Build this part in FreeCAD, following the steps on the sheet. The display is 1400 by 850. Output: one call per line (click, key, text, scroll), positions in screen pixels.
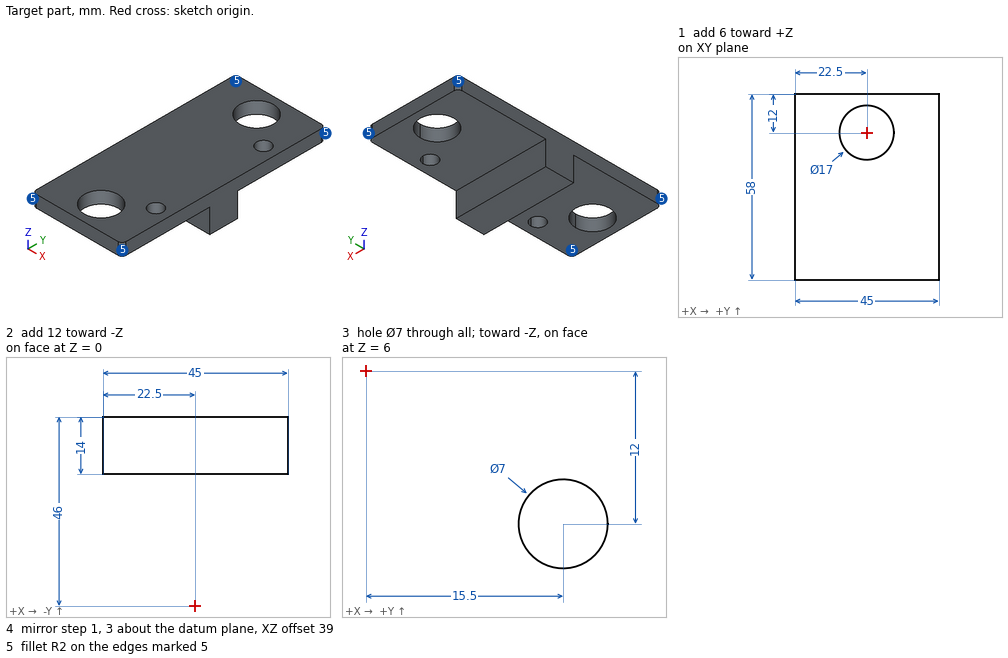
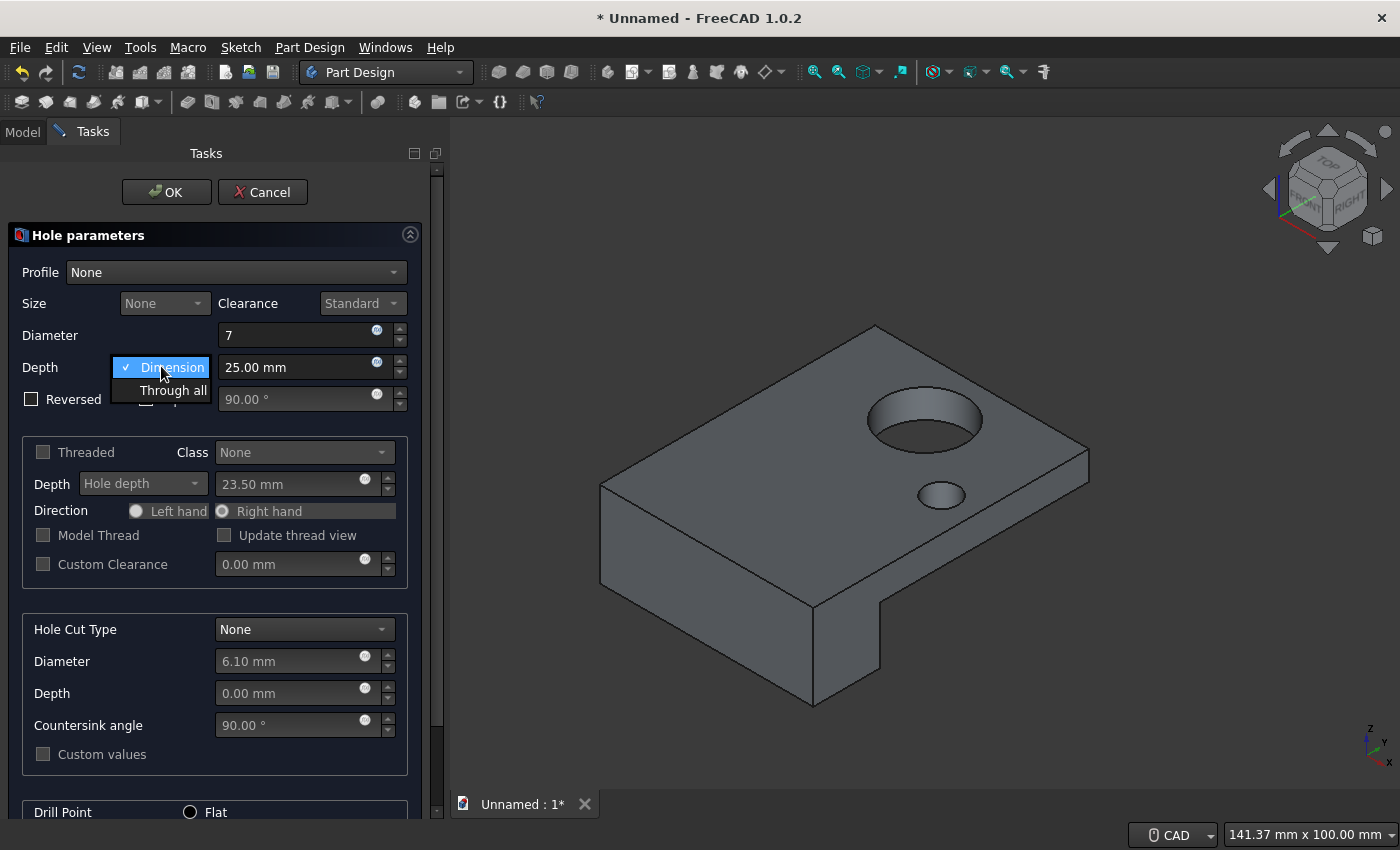
click(160, 390)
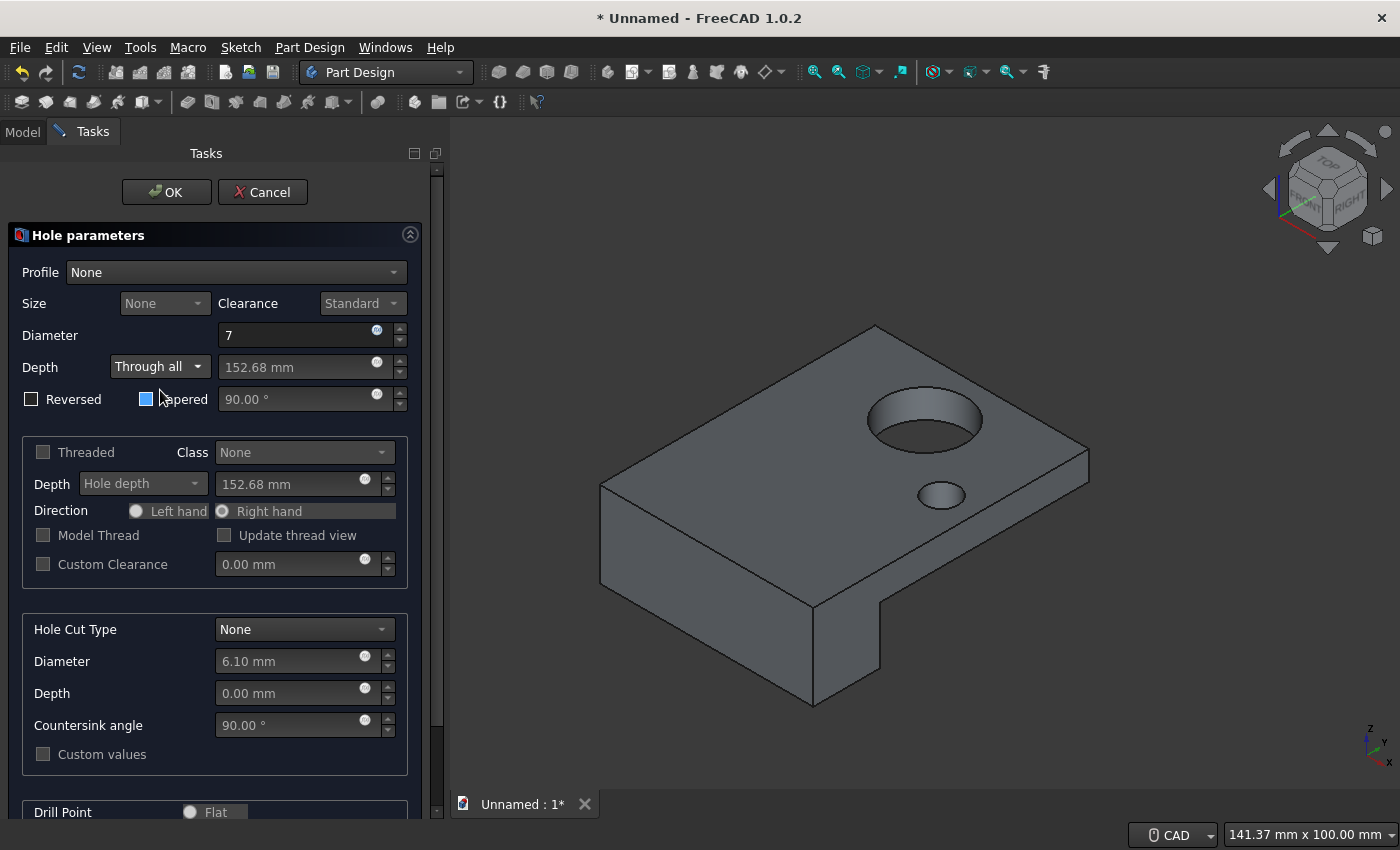
click(167, 192)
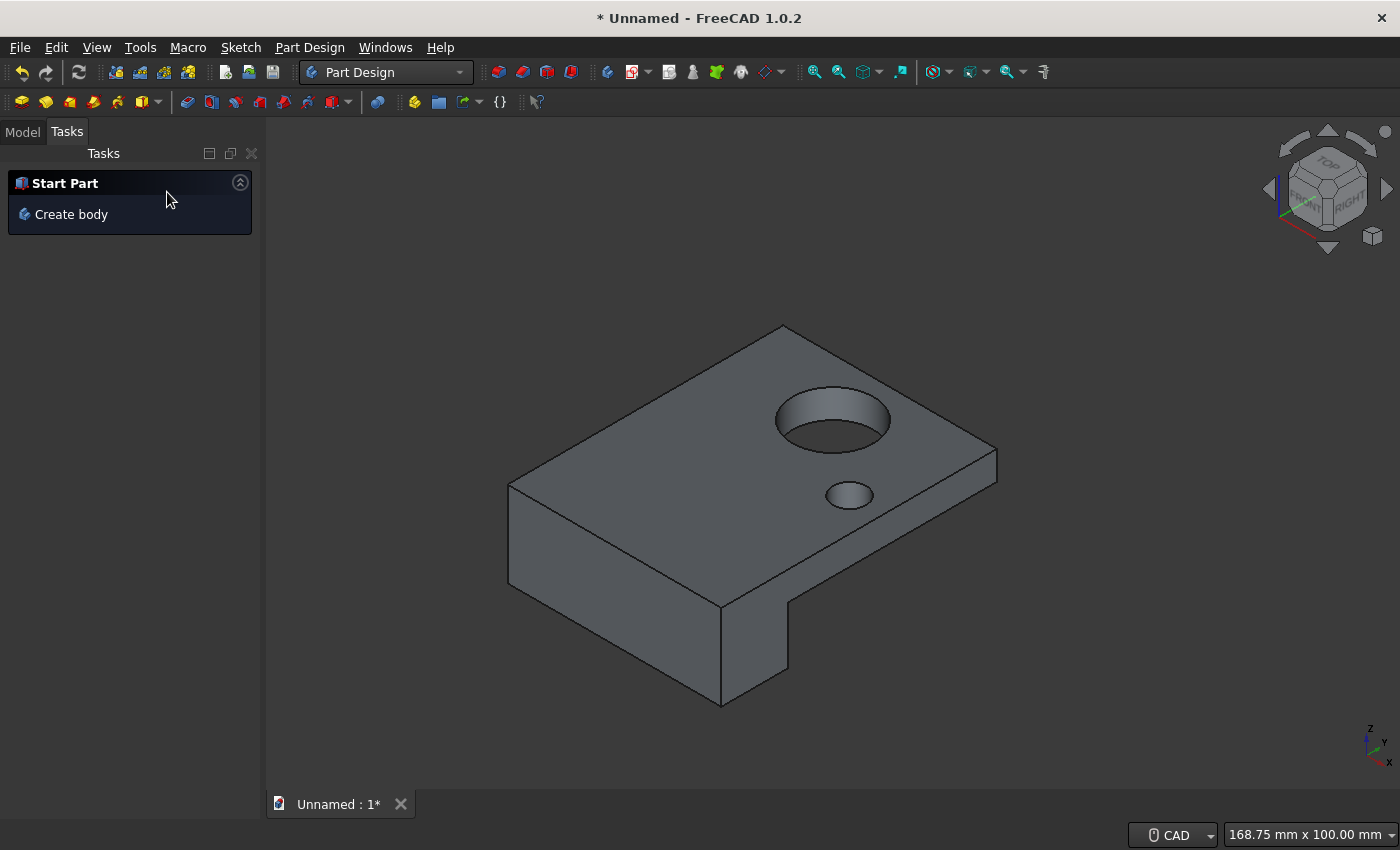
click(23, 131)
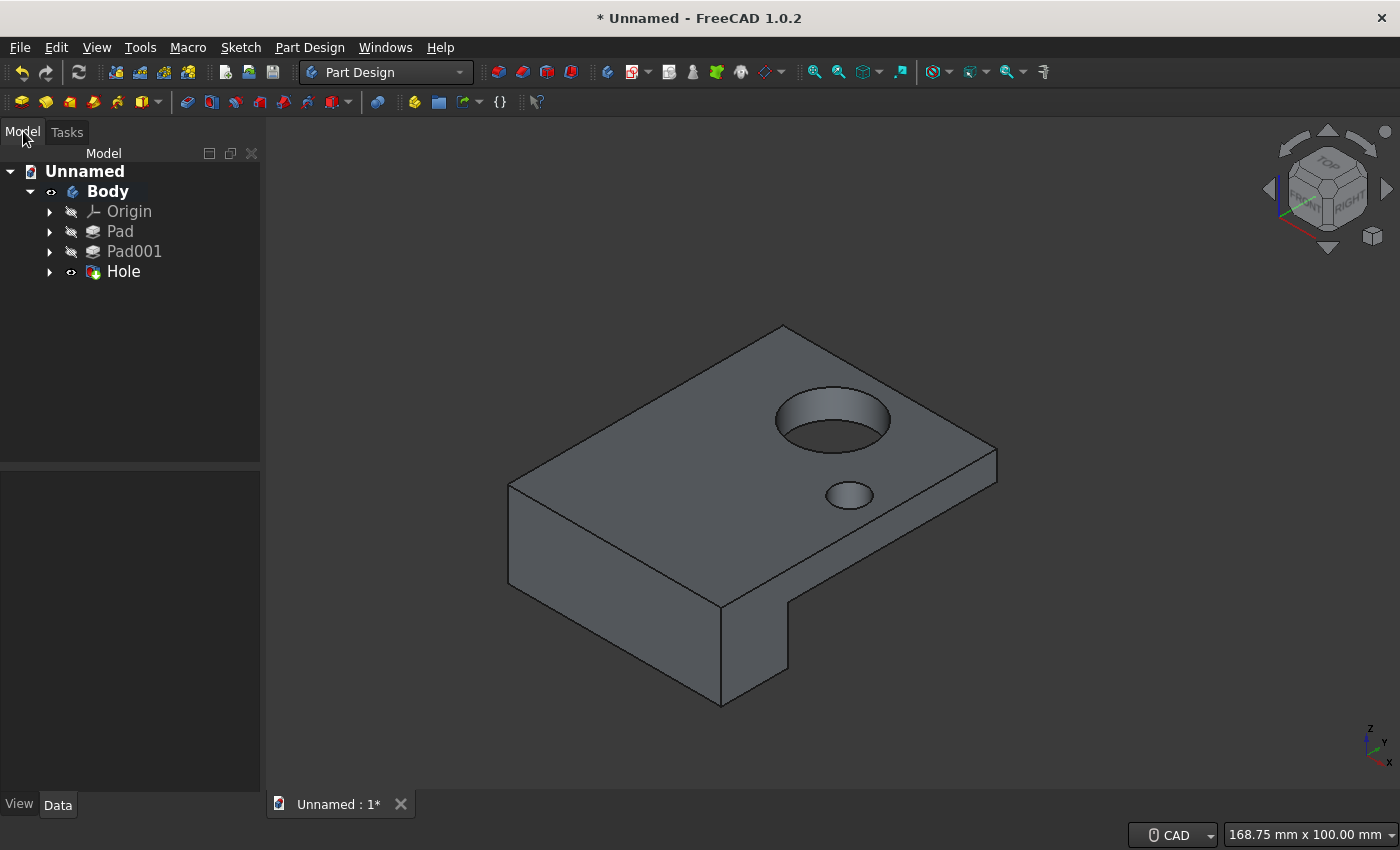
click(50, 212)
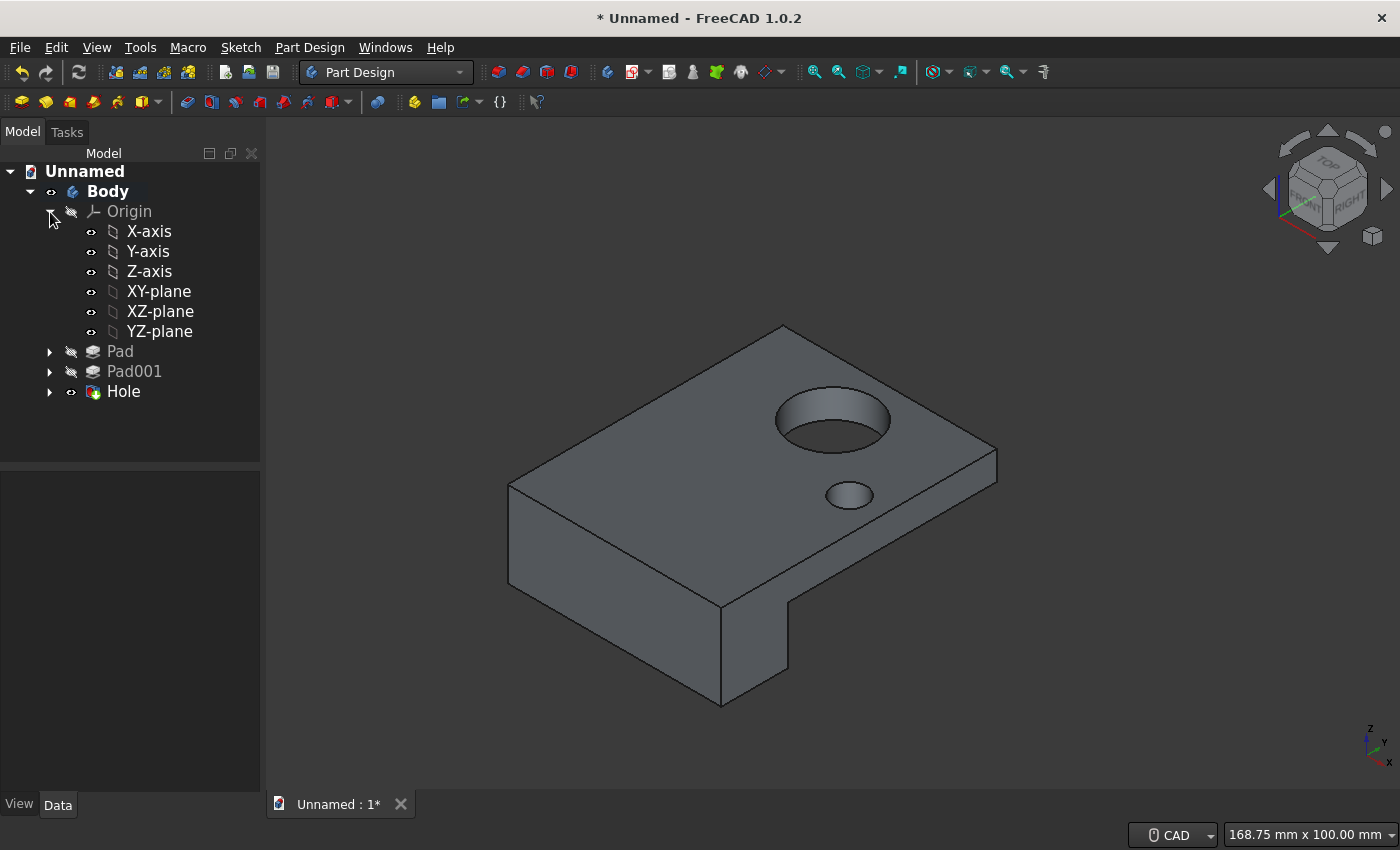
click(136, 312)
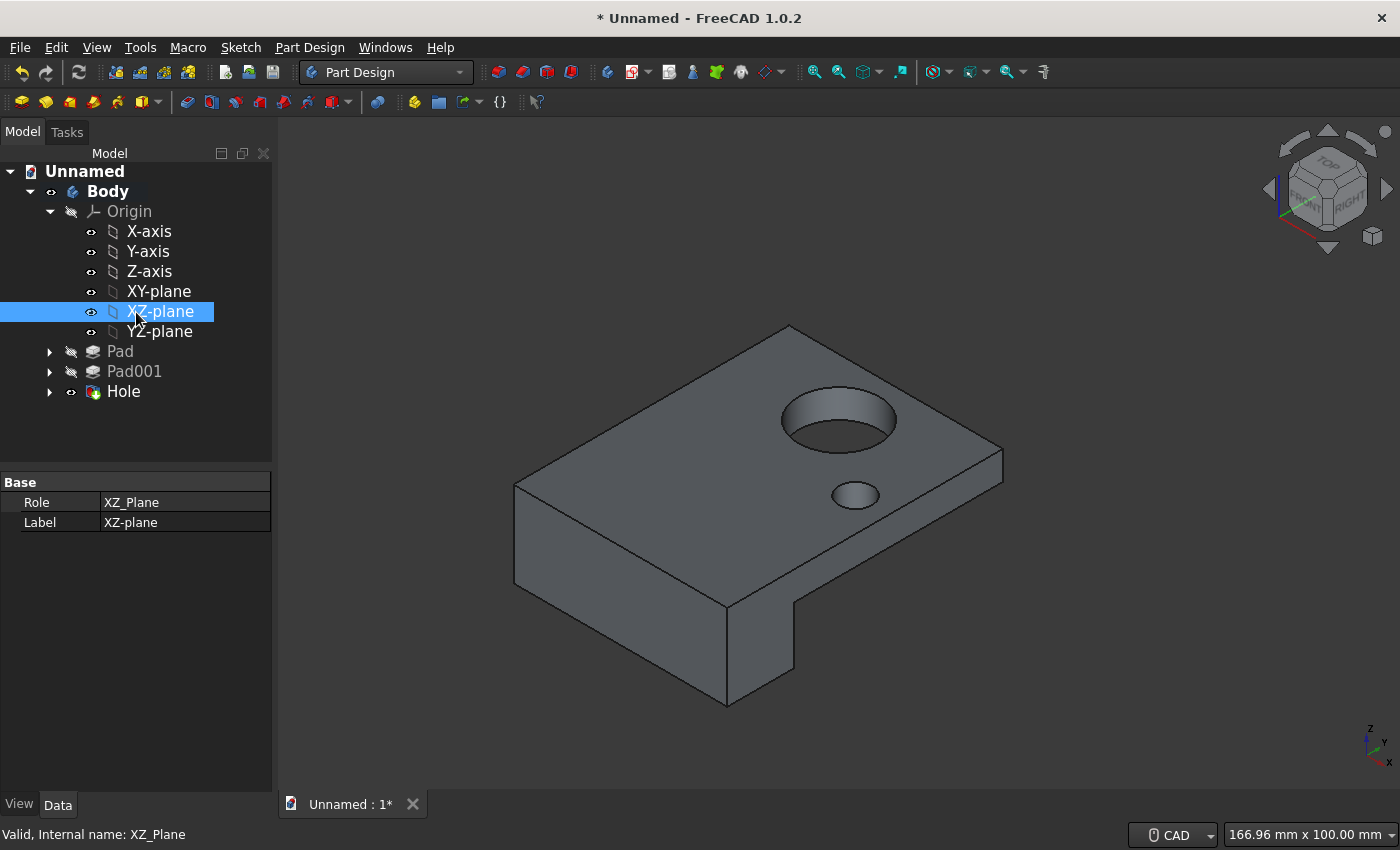
click(766, 72)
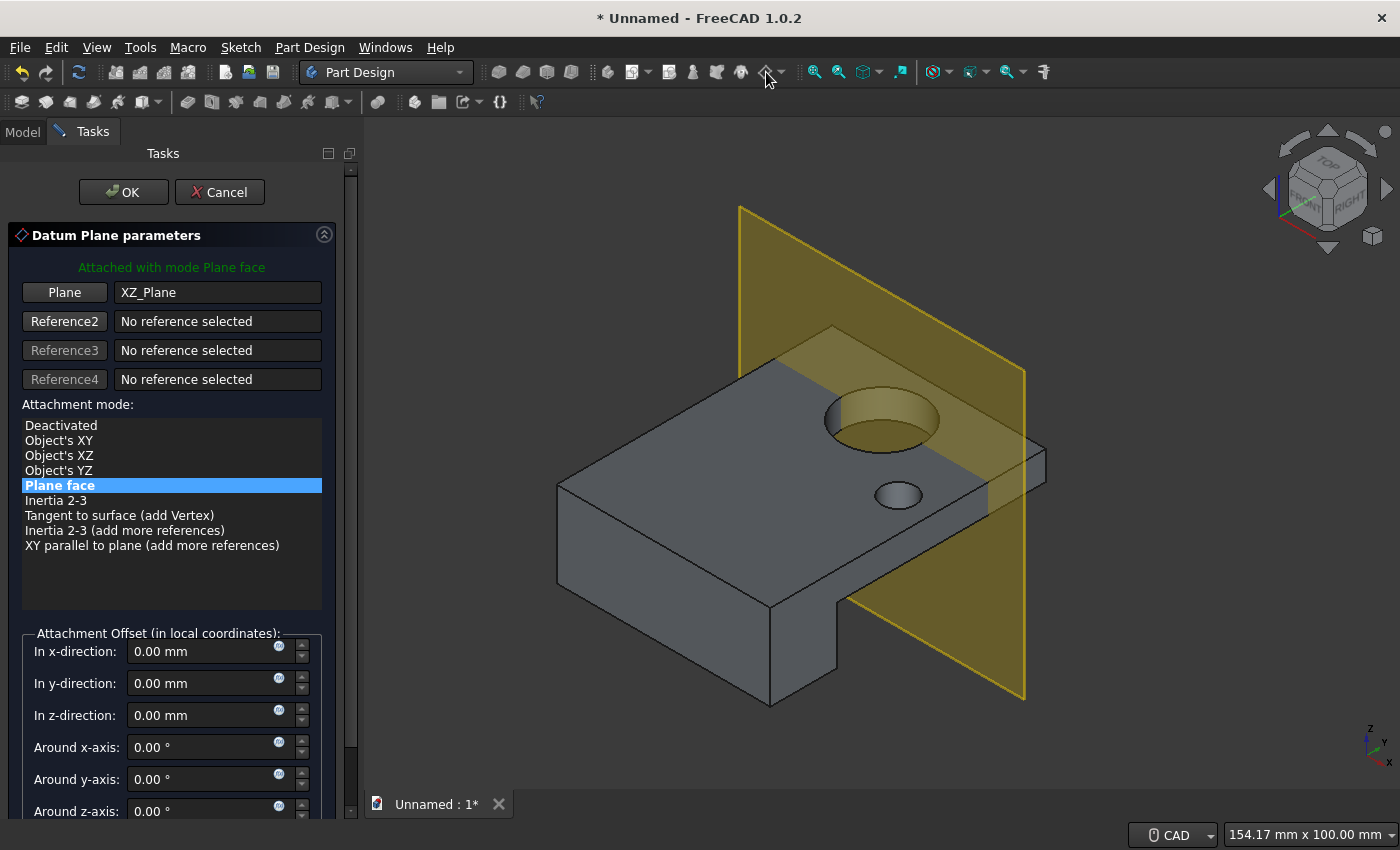
triple_click(210, 715)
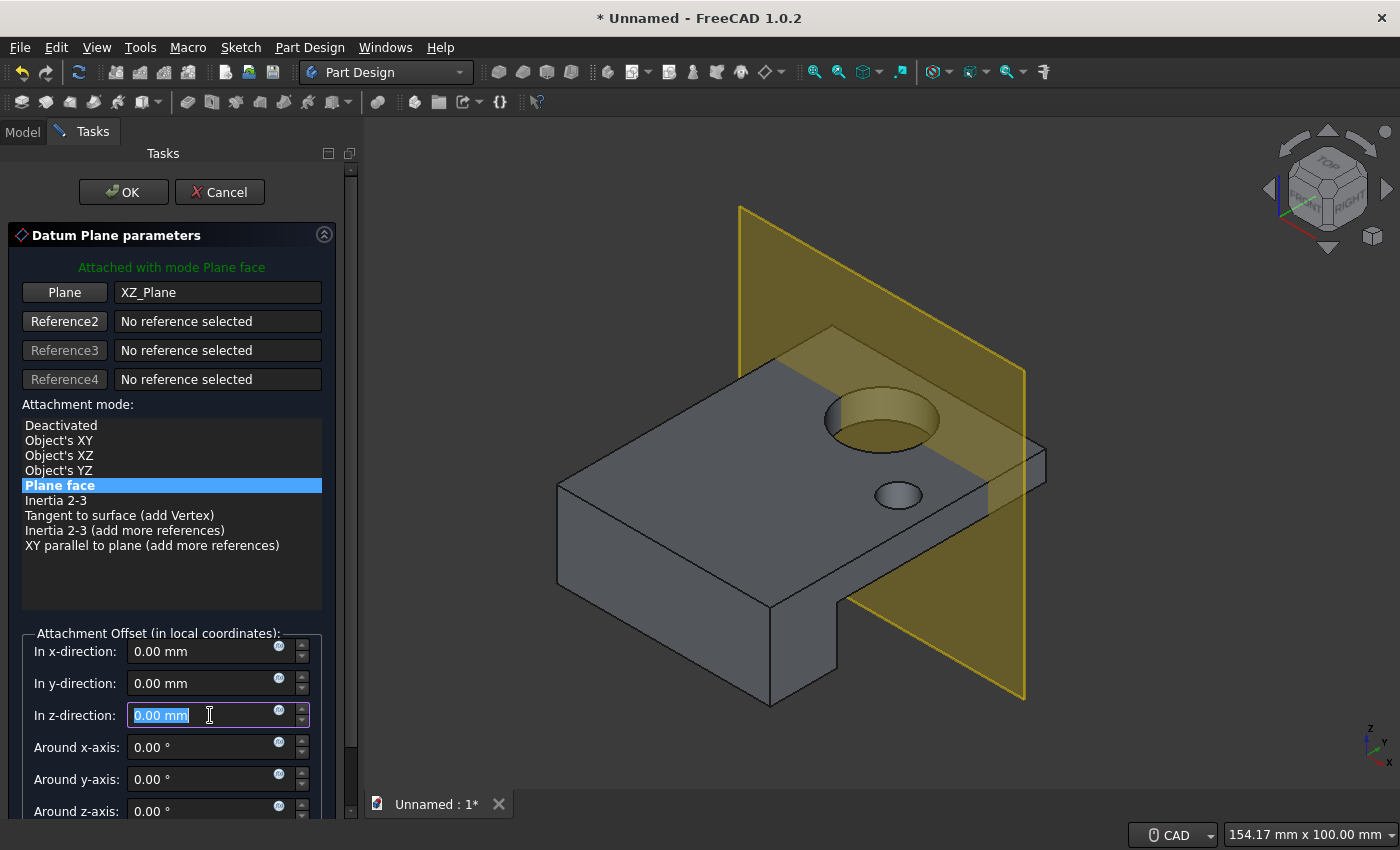
text(39)
key(Tab)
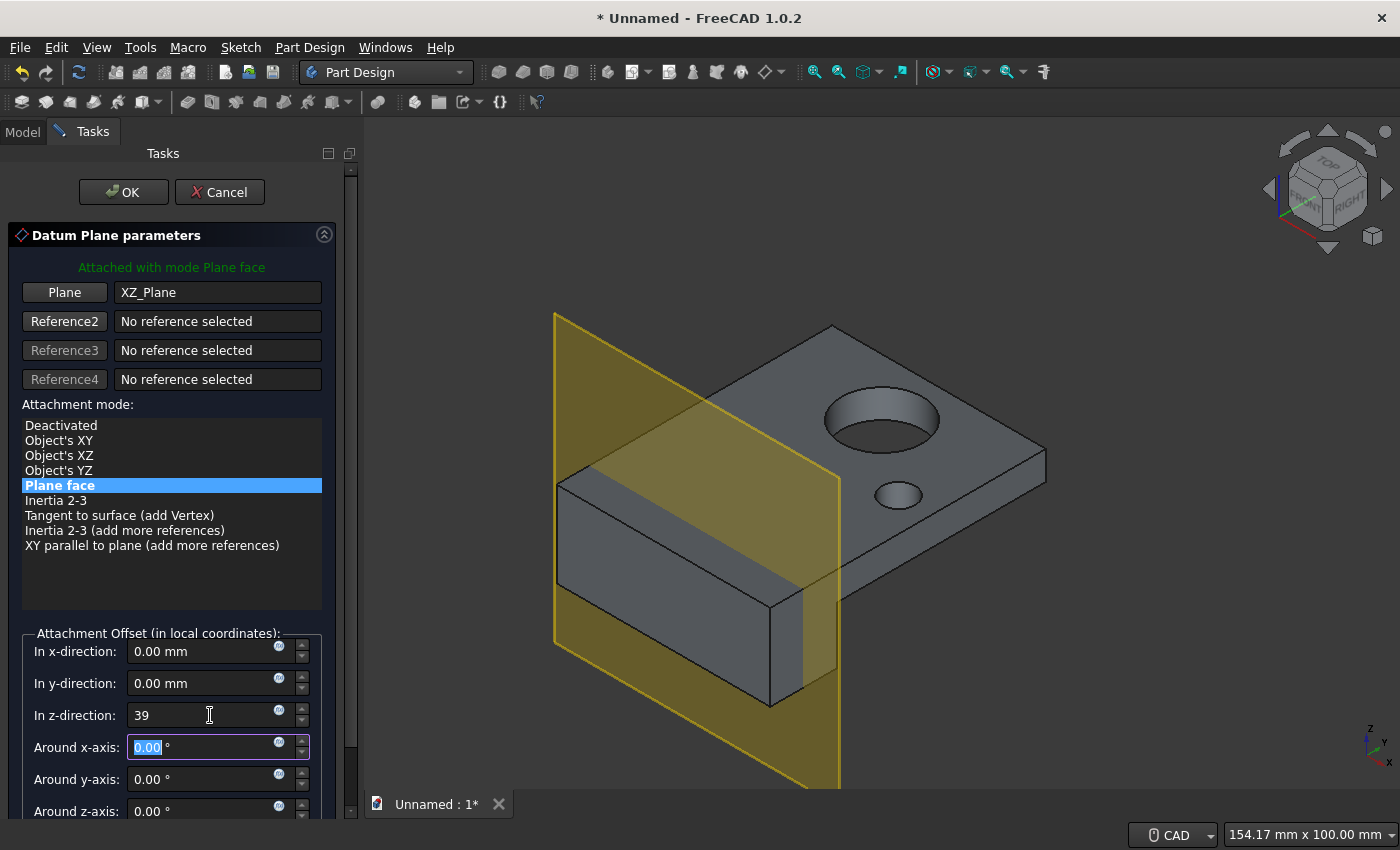
click(124, 192)